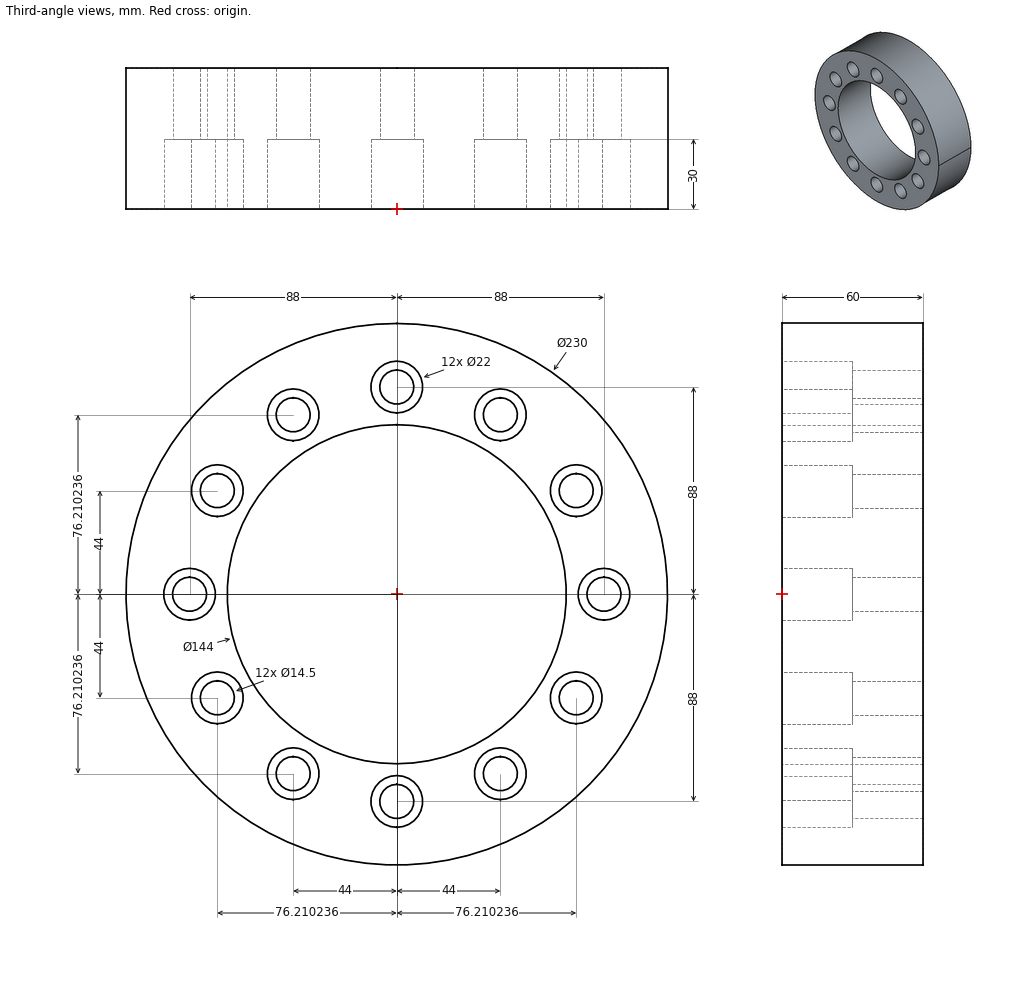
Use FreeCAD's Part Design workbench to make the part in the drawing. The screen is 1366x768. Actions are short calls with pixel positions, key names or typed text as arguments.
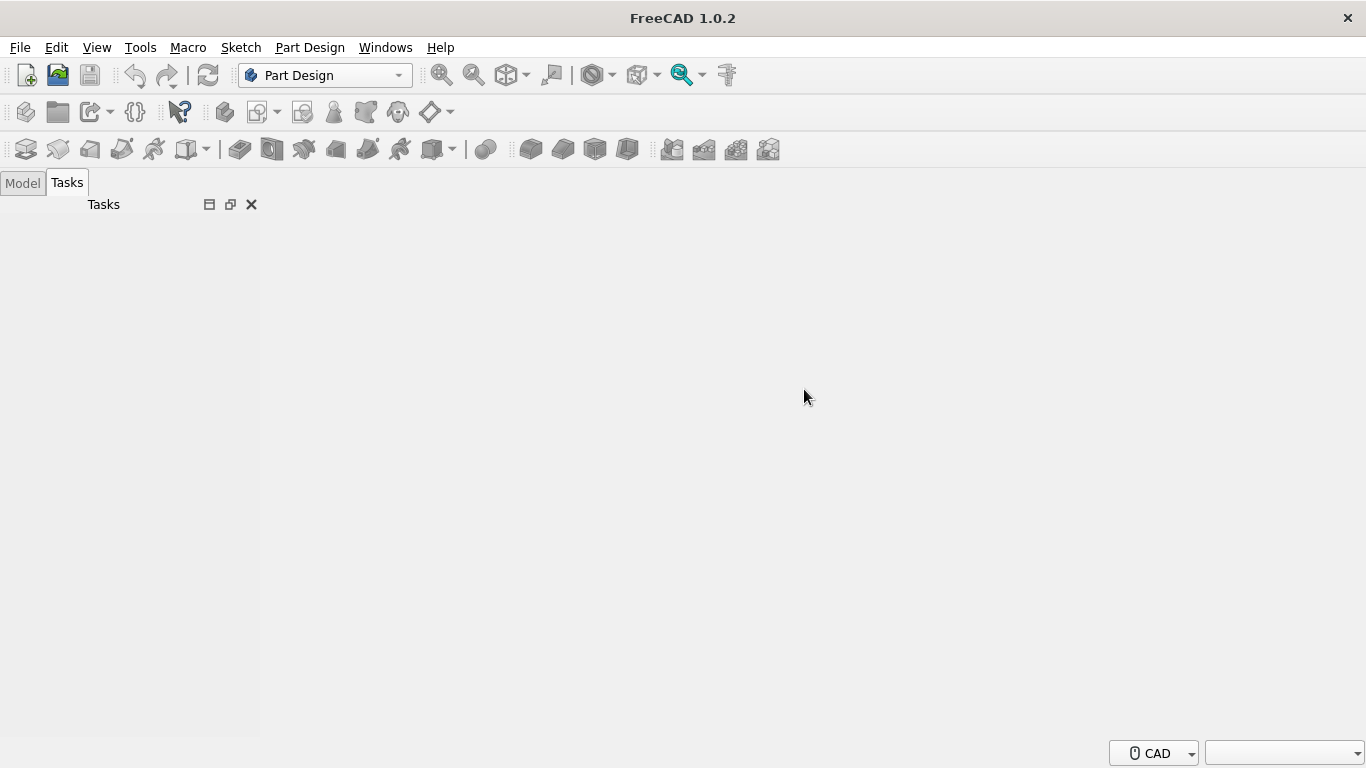
click(26, 76)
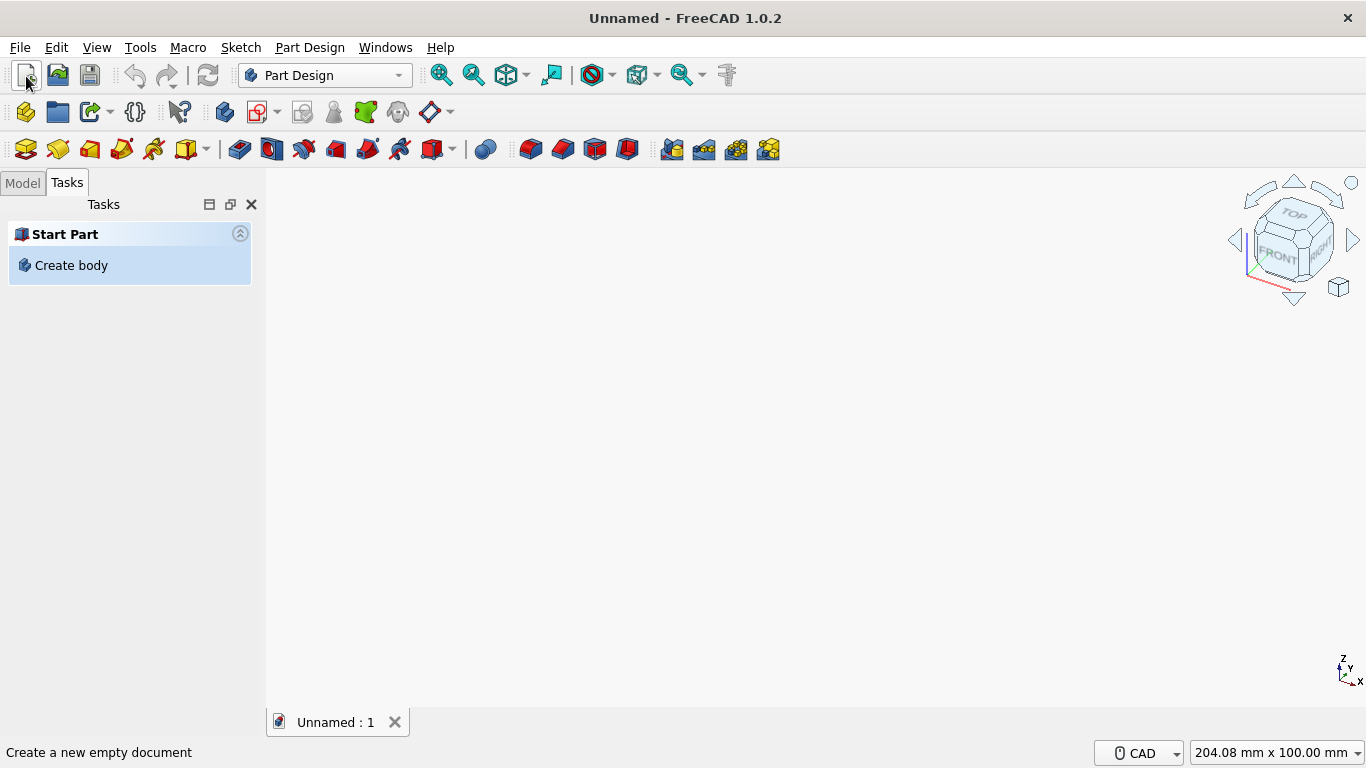
click(258, 112)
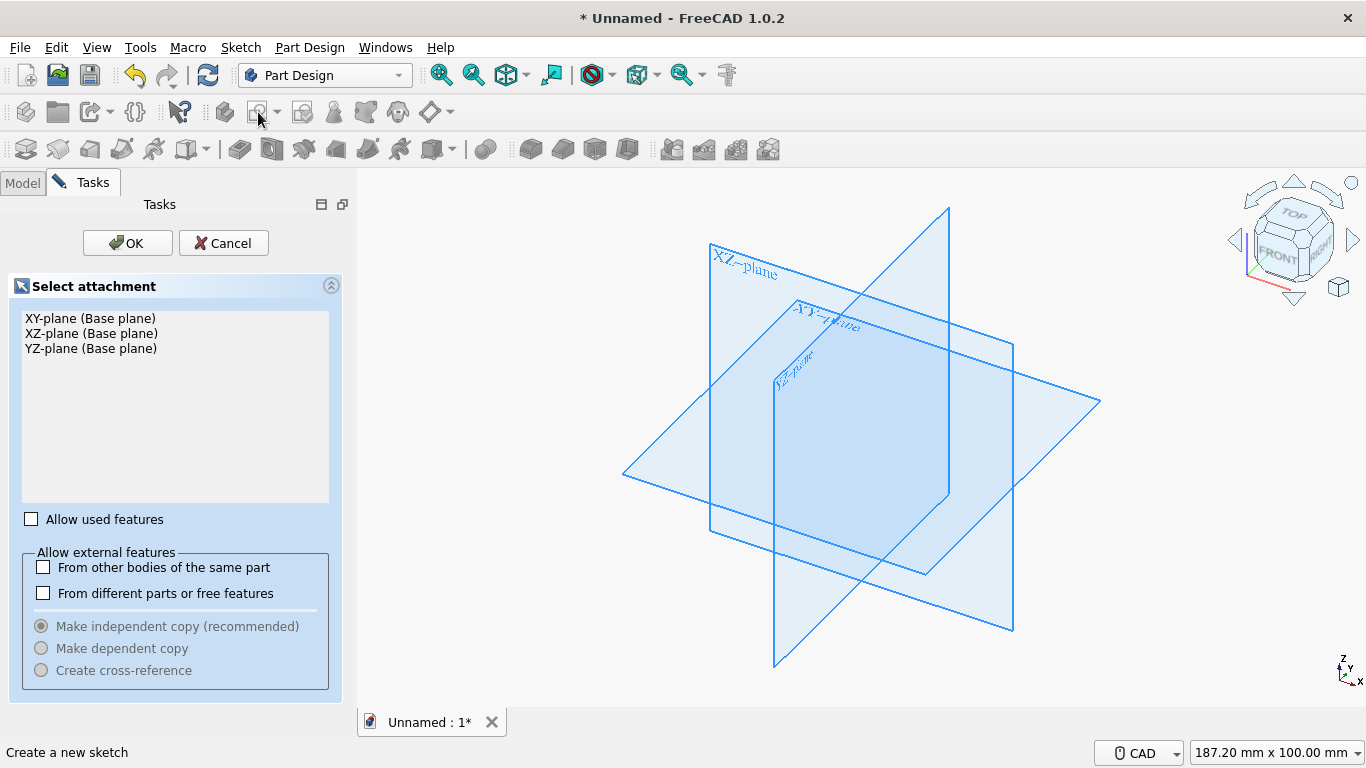
click(82, 334)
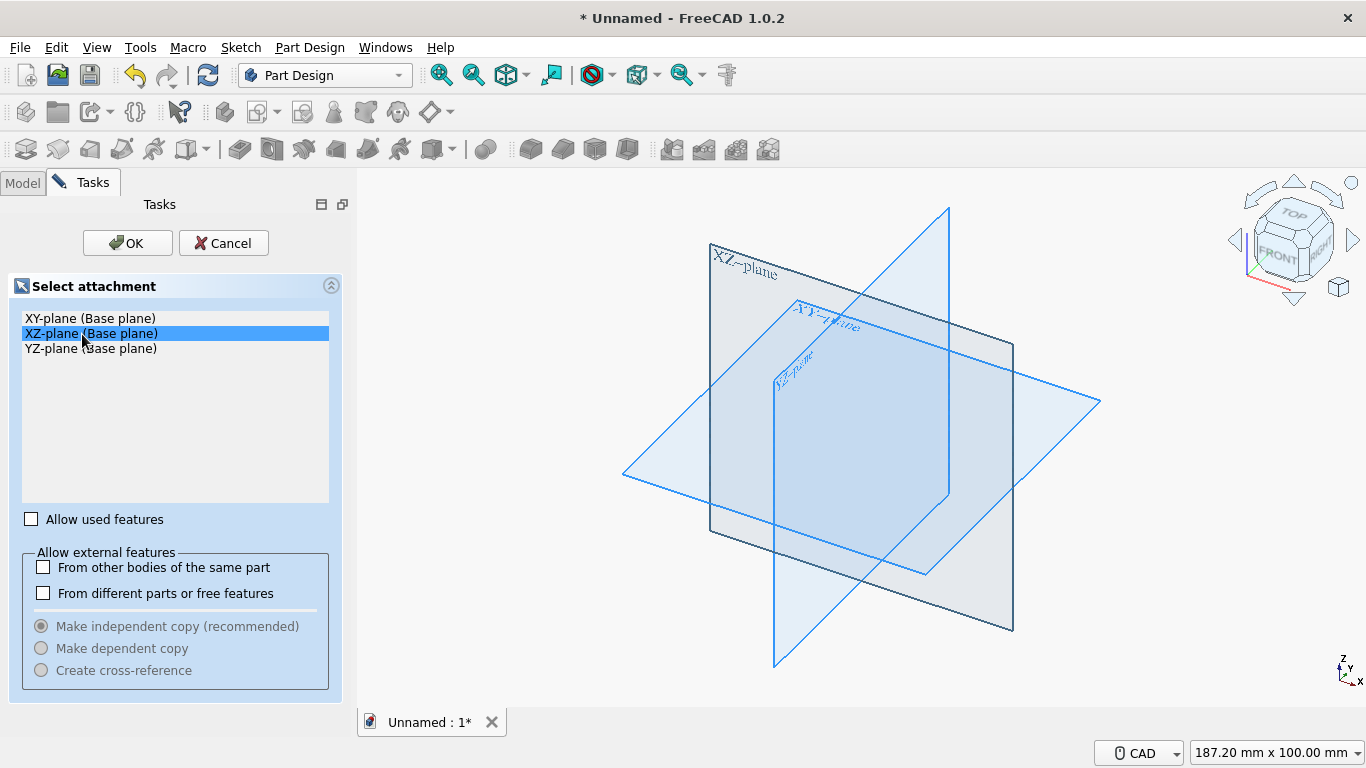
click(128, 243)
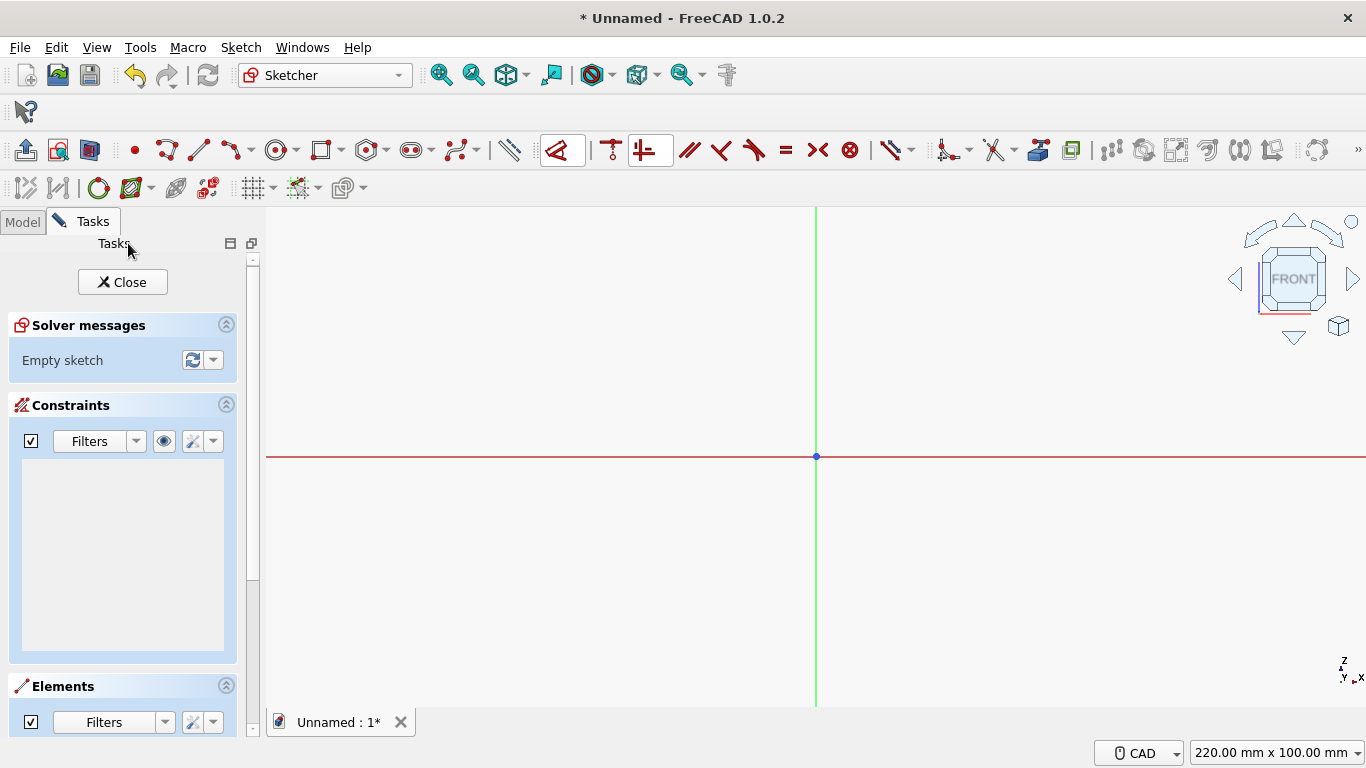
scroll(725, 457, down, 7)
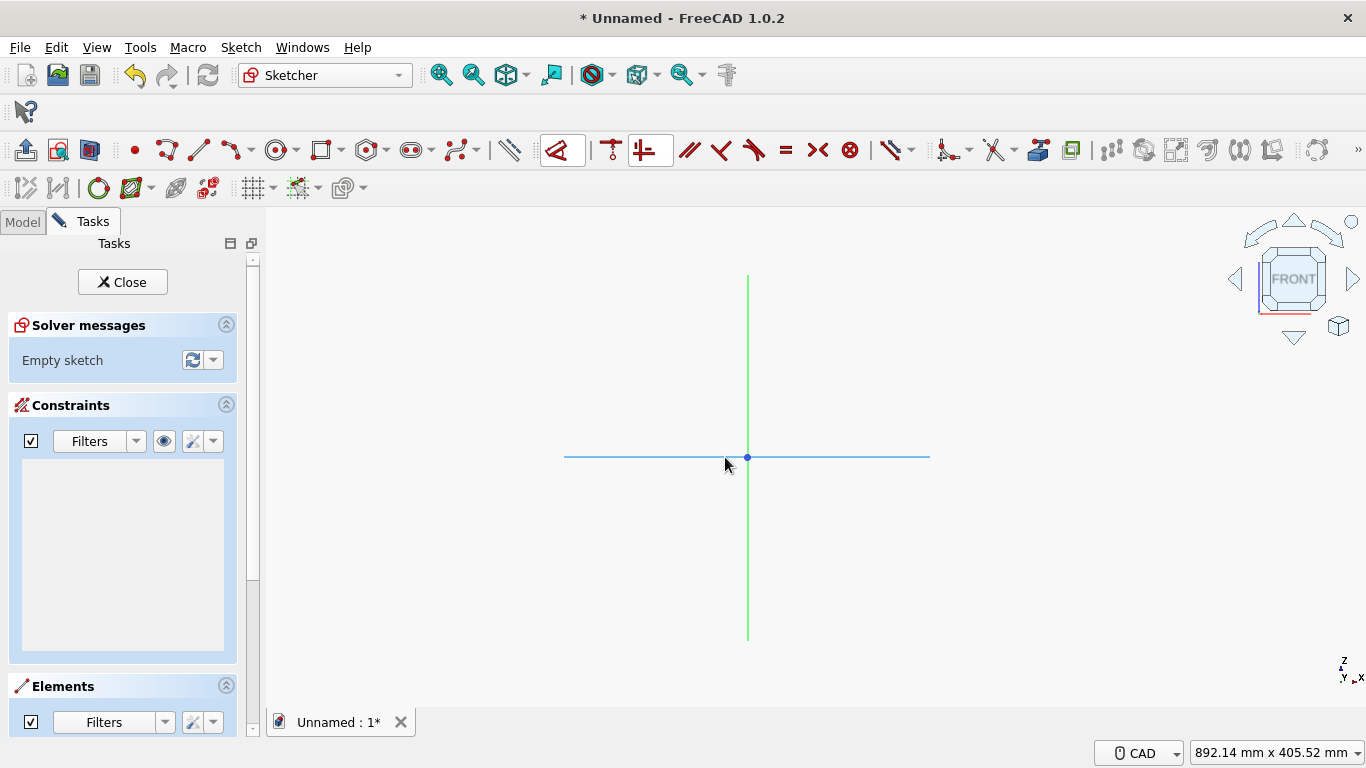
click(276, 150)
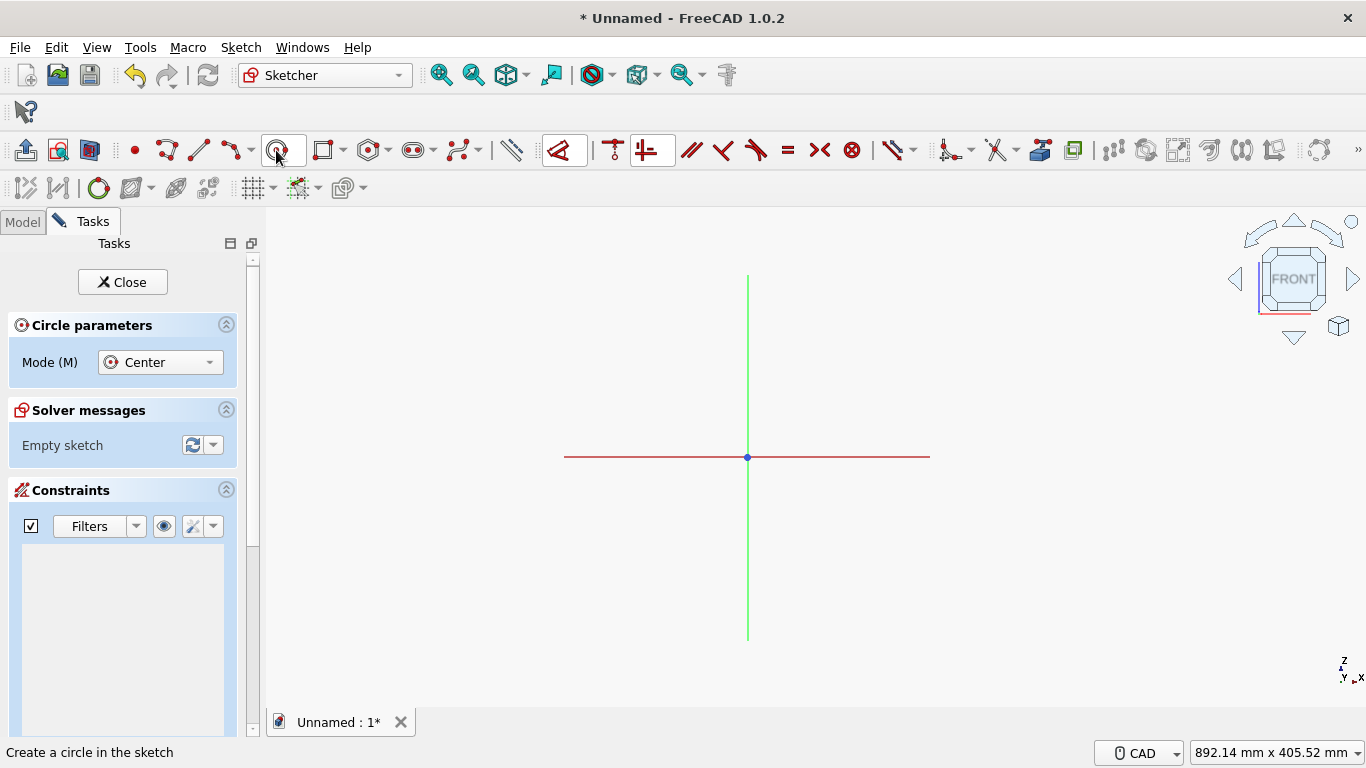
click(748, 457)
move(848, 357)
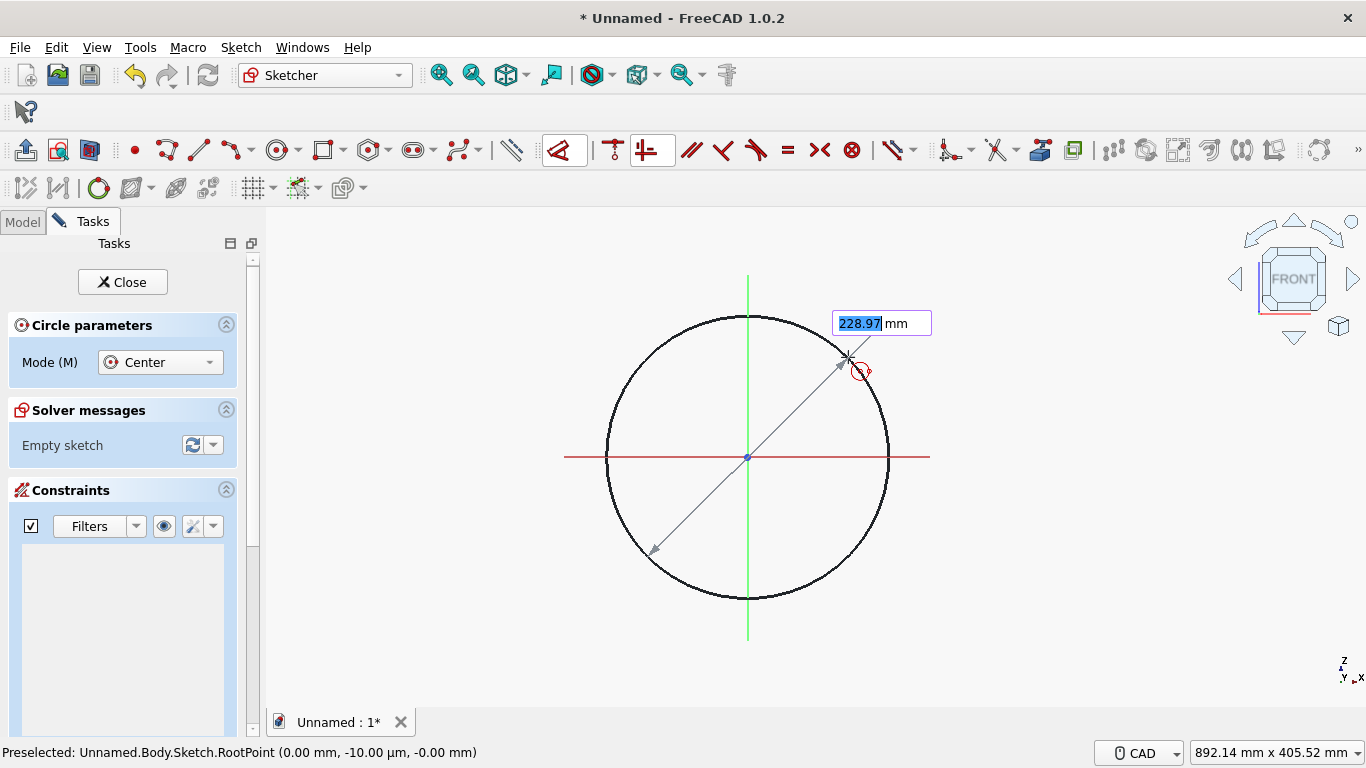
text(230)
key(Return)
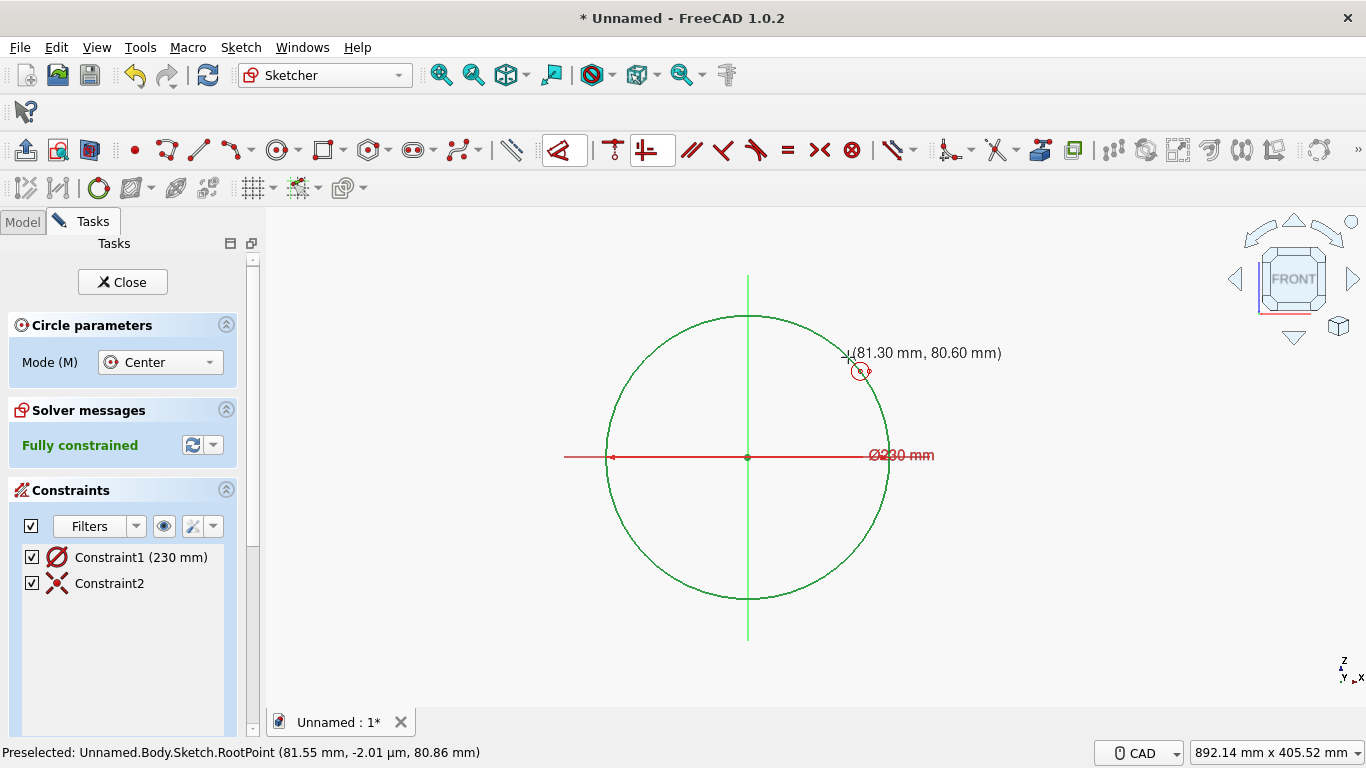
scroll(654, 512, up, 5)